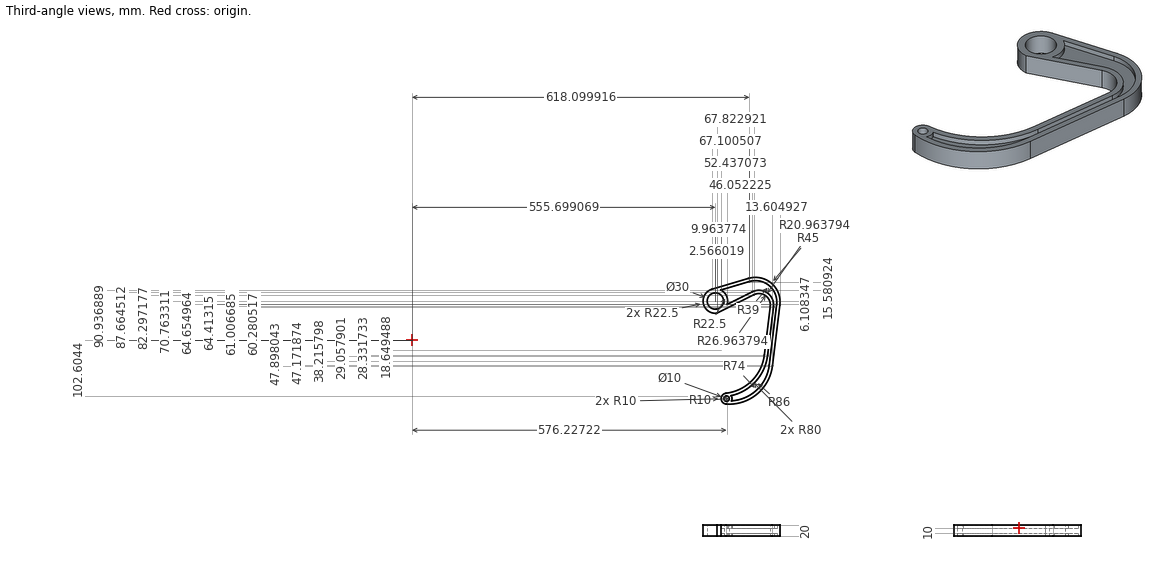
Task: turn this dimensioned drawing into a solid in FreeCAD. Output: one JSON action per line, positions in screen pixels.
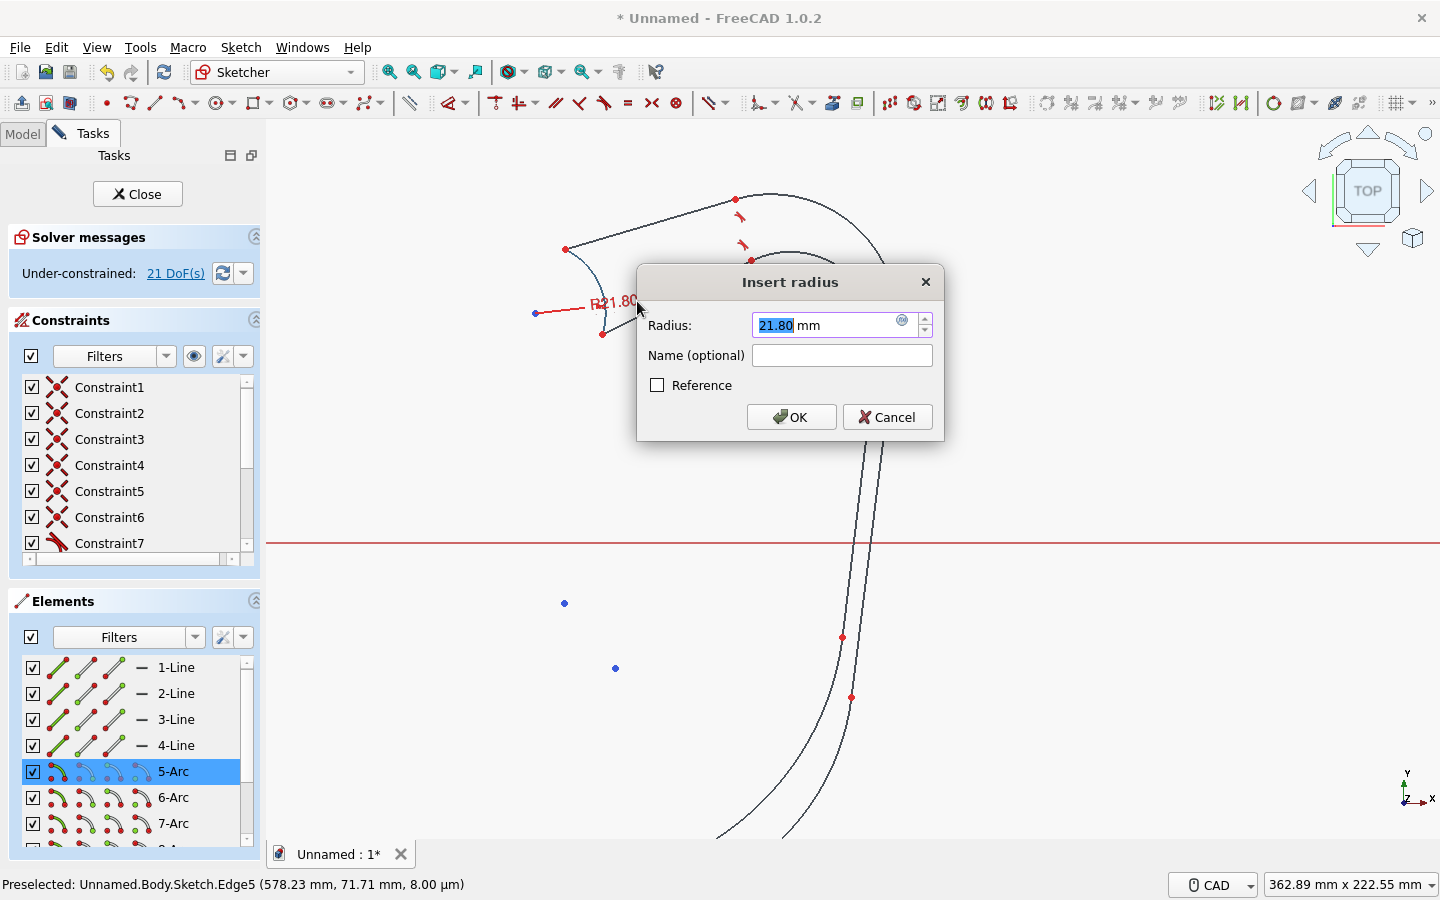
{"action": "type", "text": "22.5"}
{"action": "key", "text": "Return"}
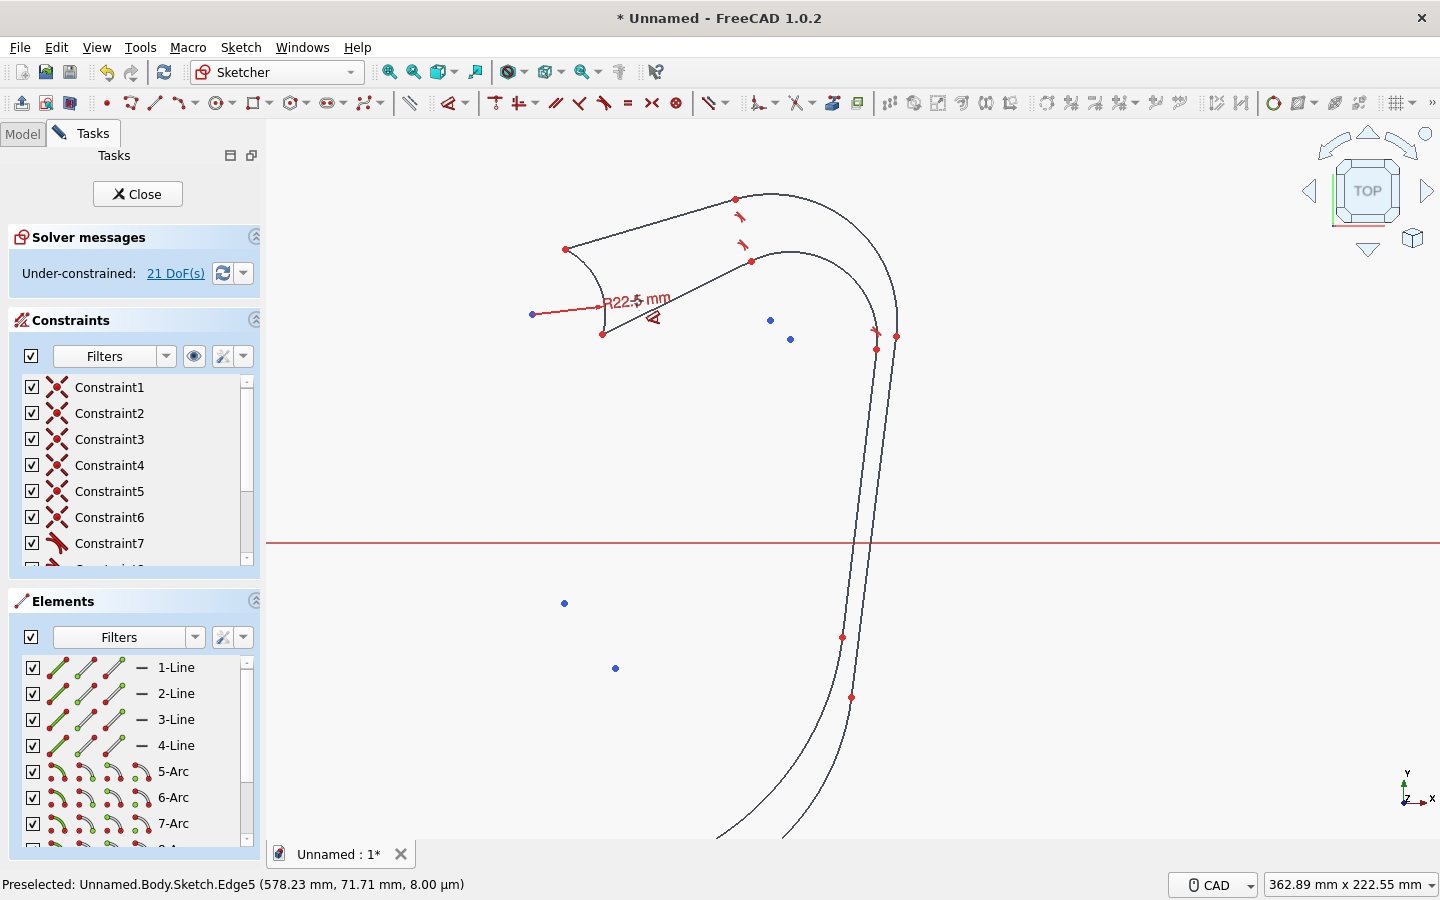
{"action": "left_click", "coordinate": [866, 295]}
{"action": "left_click", "coordinate": [910, 336]}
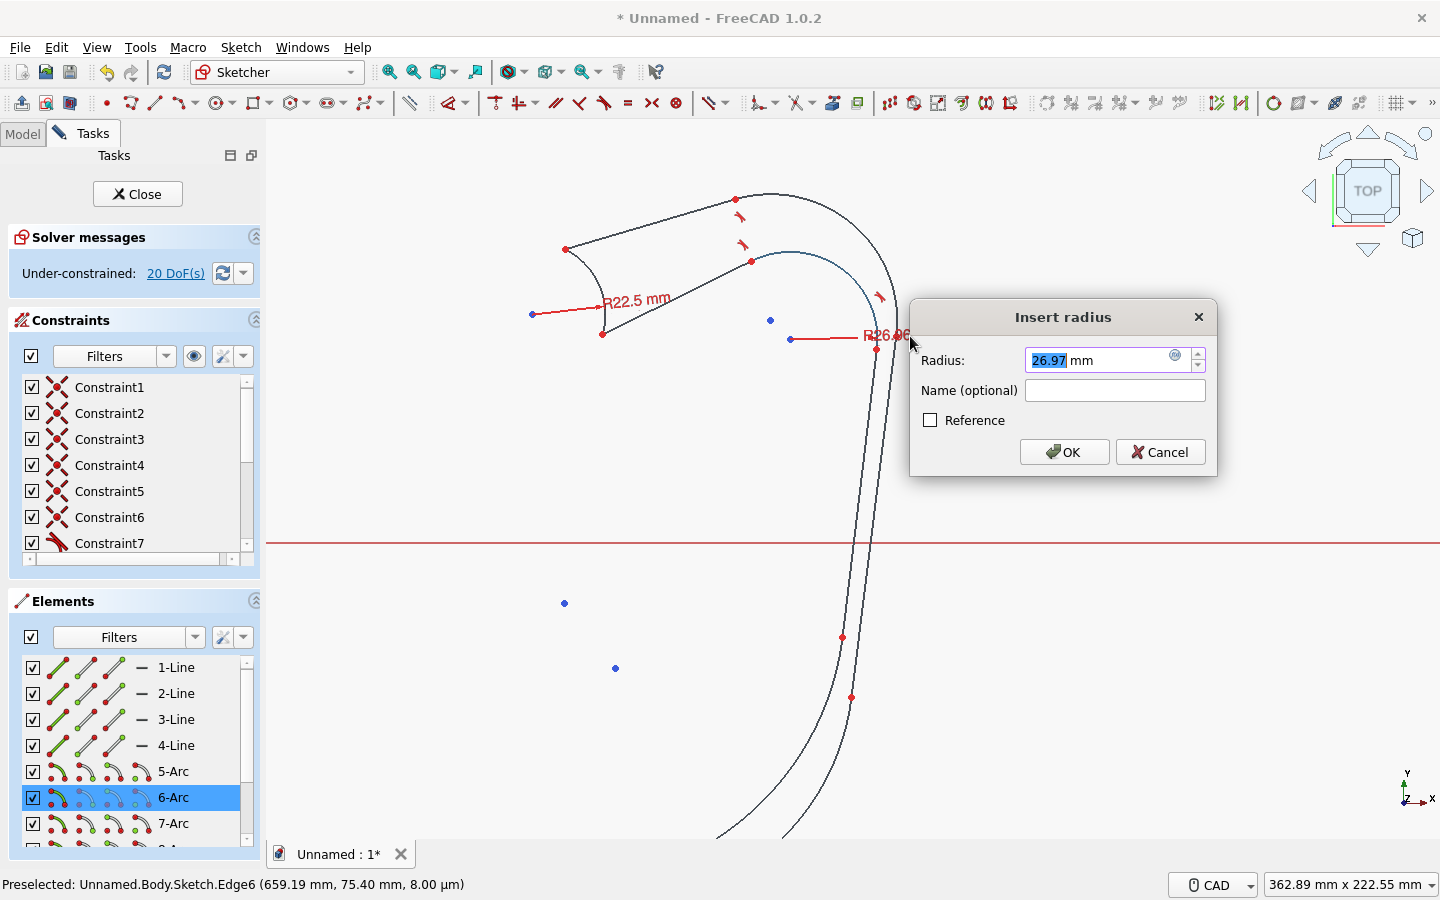
{"action": "type", "text": "26.963794"}
{"action": "key", "text": "Return"}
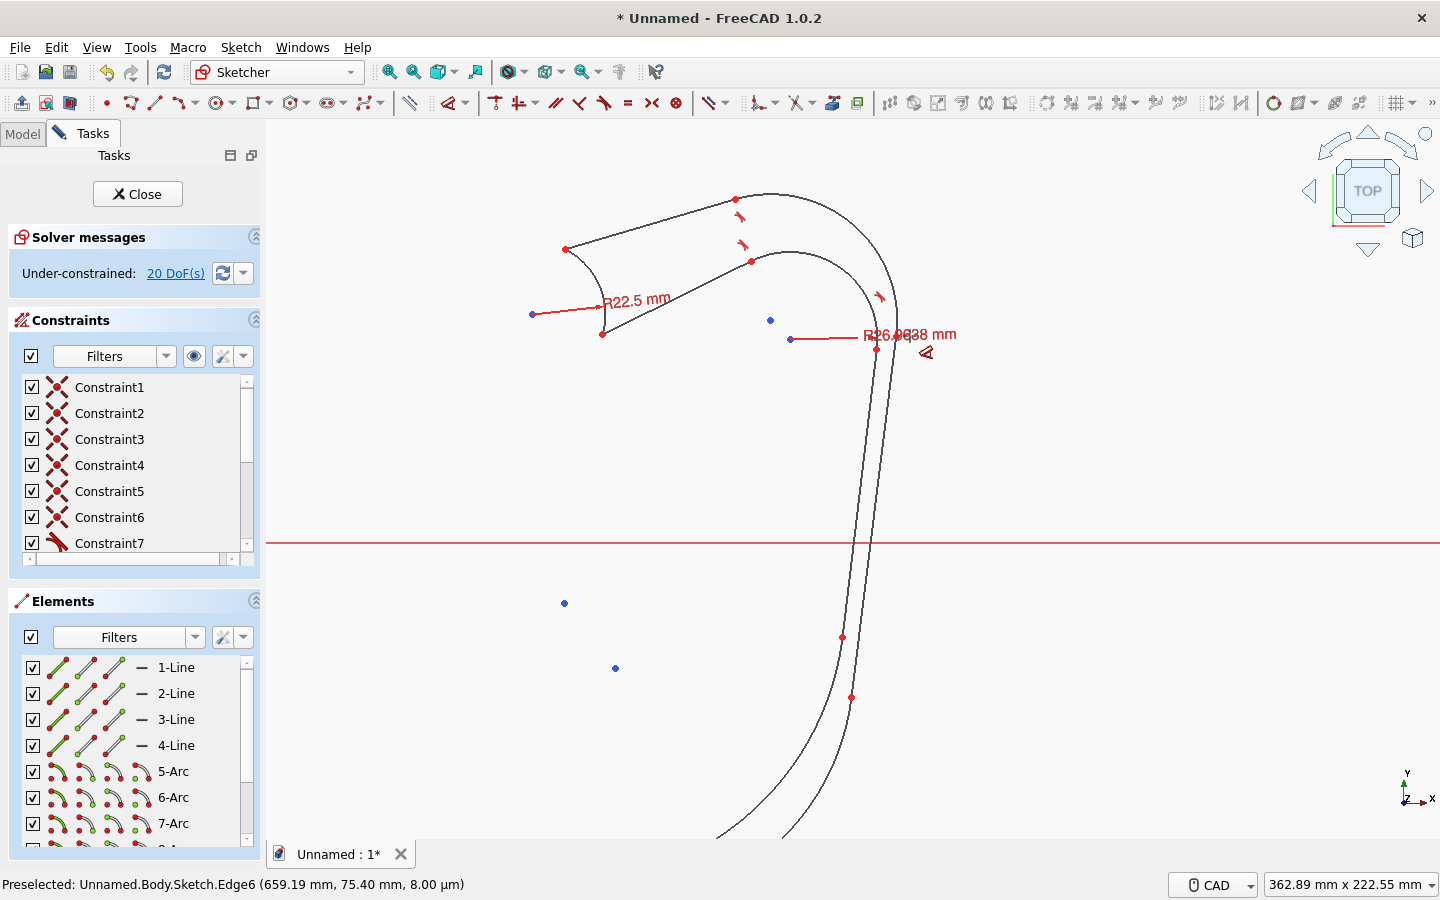
{"action": "left_click", "coordinate": [812, 735]}
{"action": "left_click", "coordinate": [877, 600]}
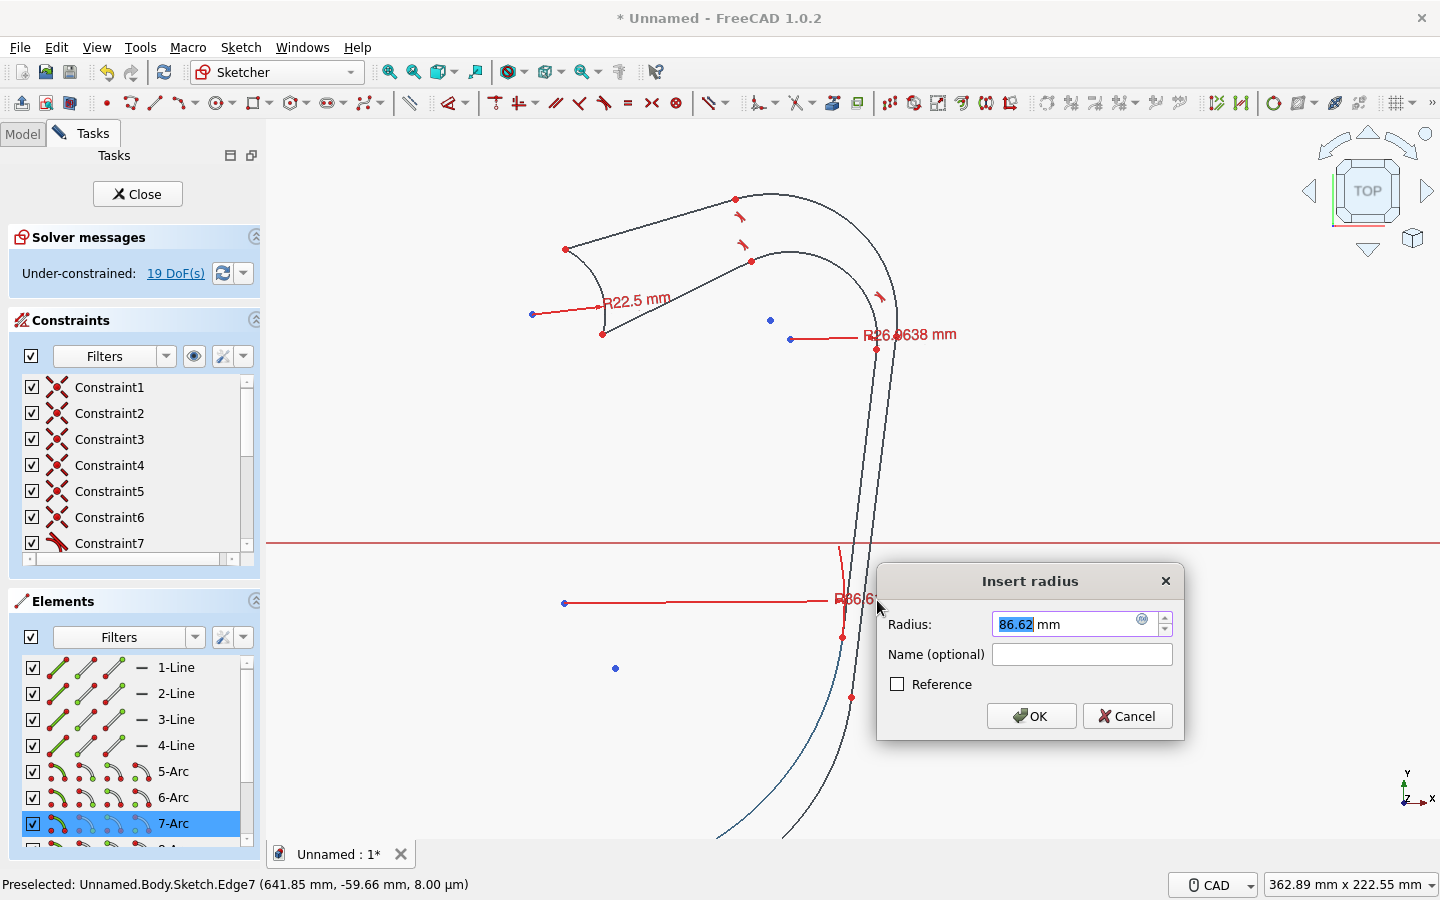
{"action": "type", "text": "86"}
{"action": "key", "text": "Return"}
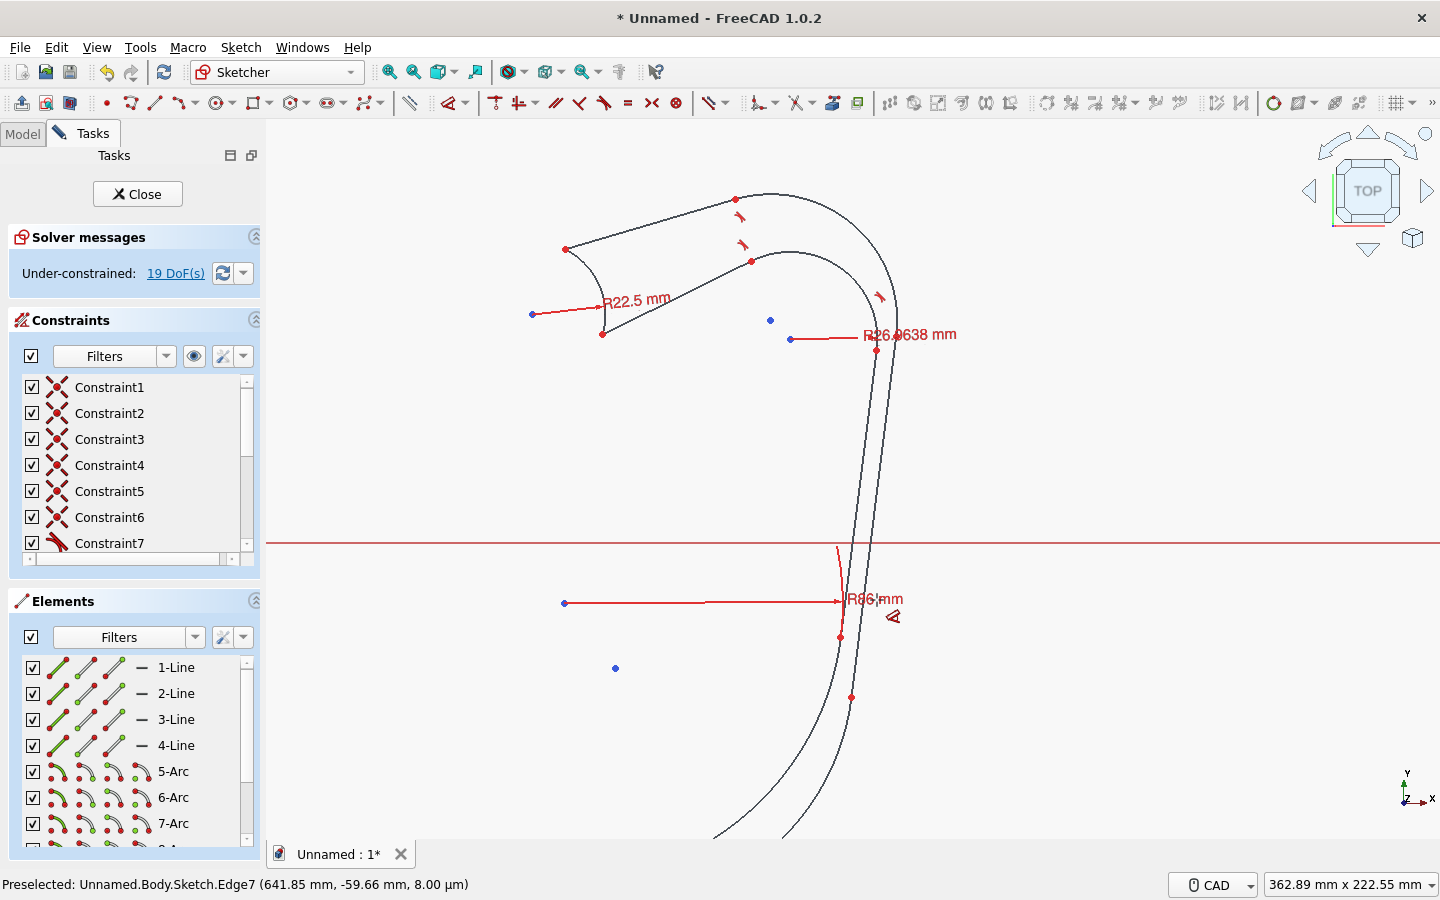
{"action": "scroll", "coordinate": [895, 331], "scroll_direction": "down", "scroll_amount": 2}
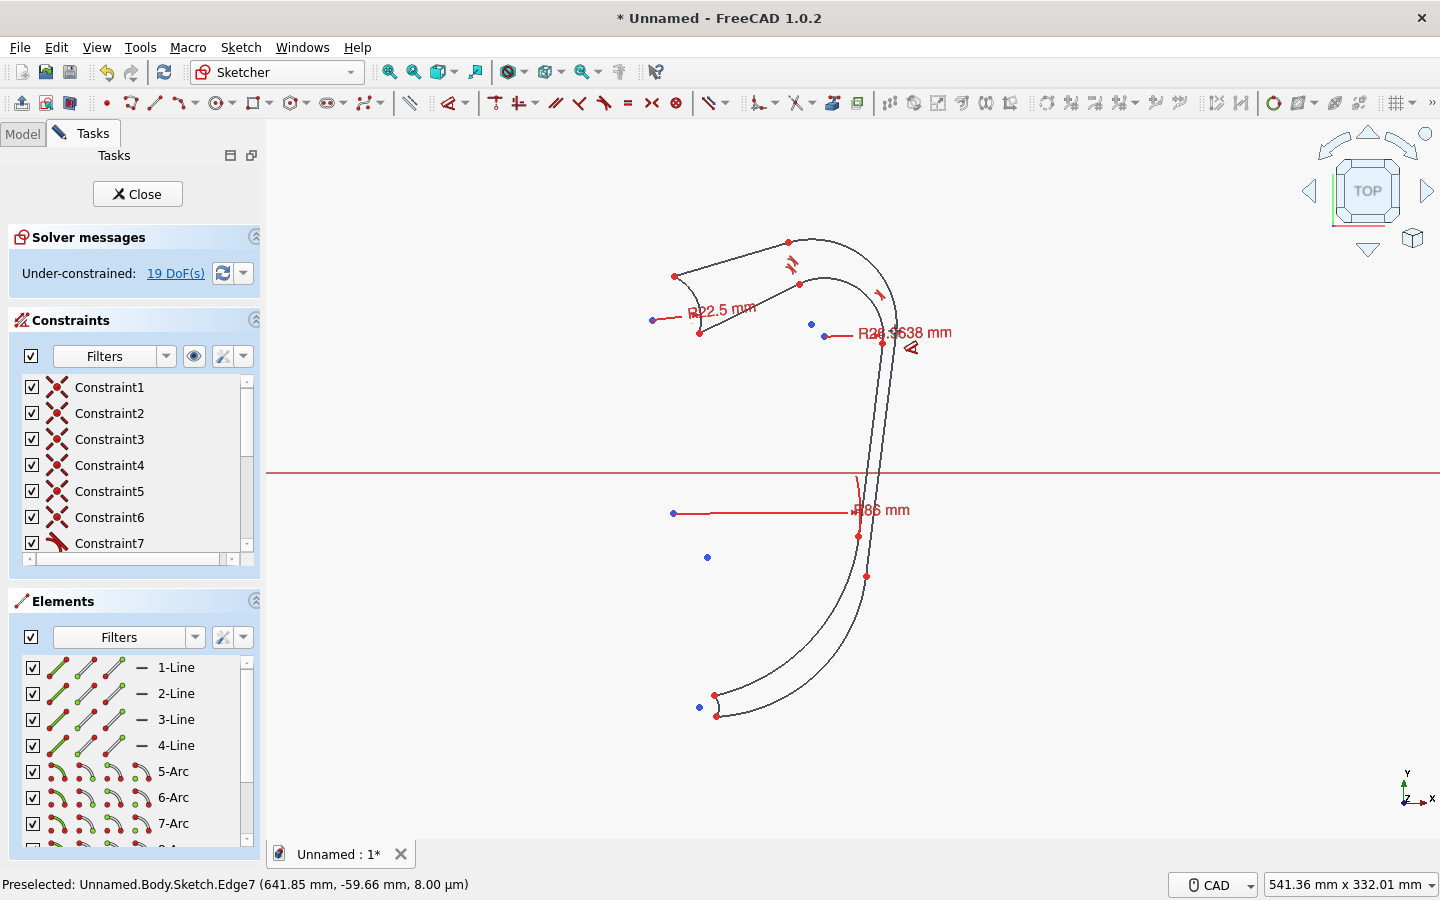
{"action": "scroll", "coordinate": [719, 710], "scroll_direction": "up", "scroll_amount": 4}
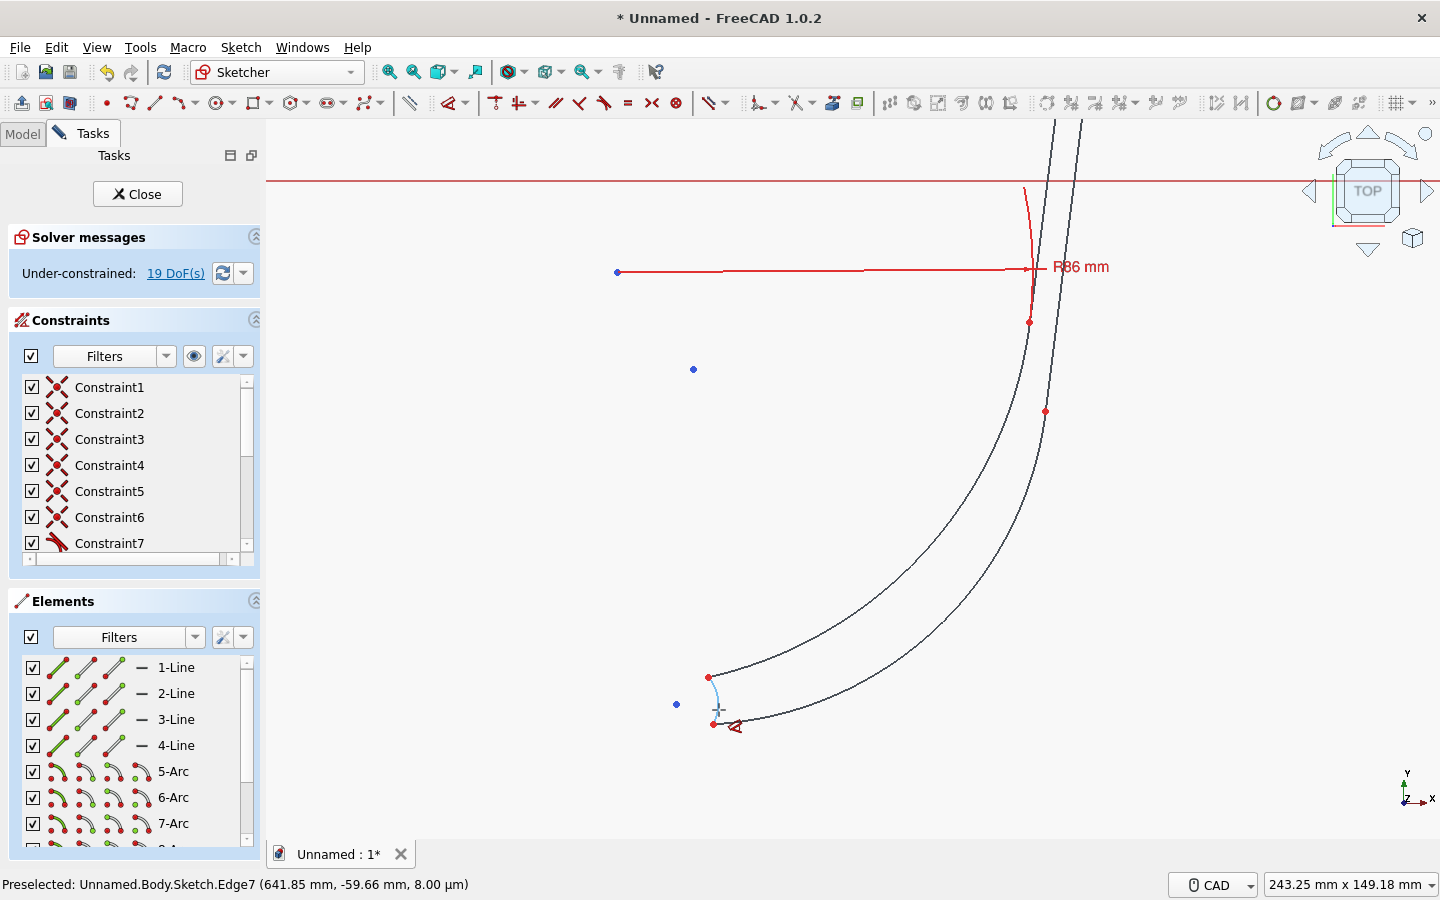
{"action": "left_click", "coordinate": [718, 710]}
{"action": "left_click", "coordinate": [736, 748]}